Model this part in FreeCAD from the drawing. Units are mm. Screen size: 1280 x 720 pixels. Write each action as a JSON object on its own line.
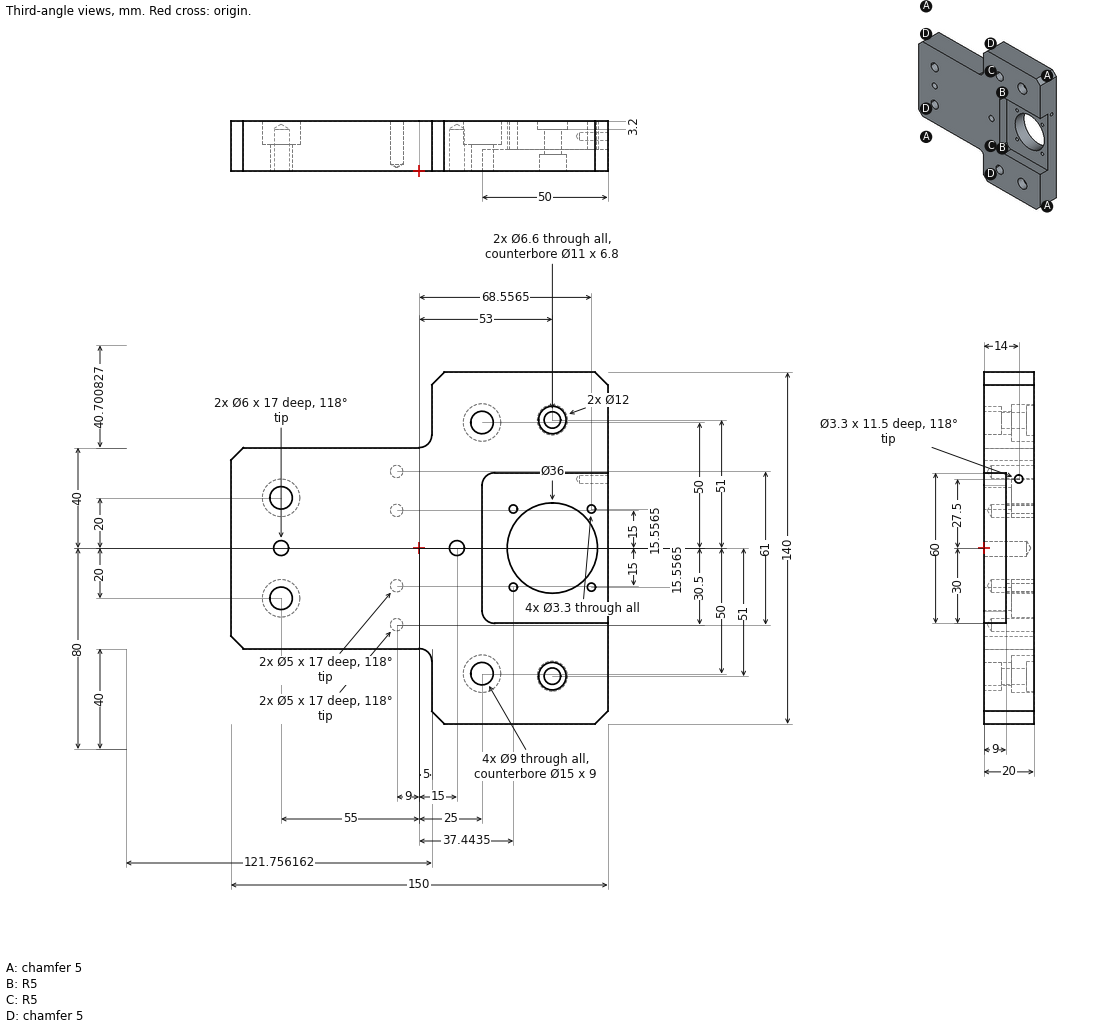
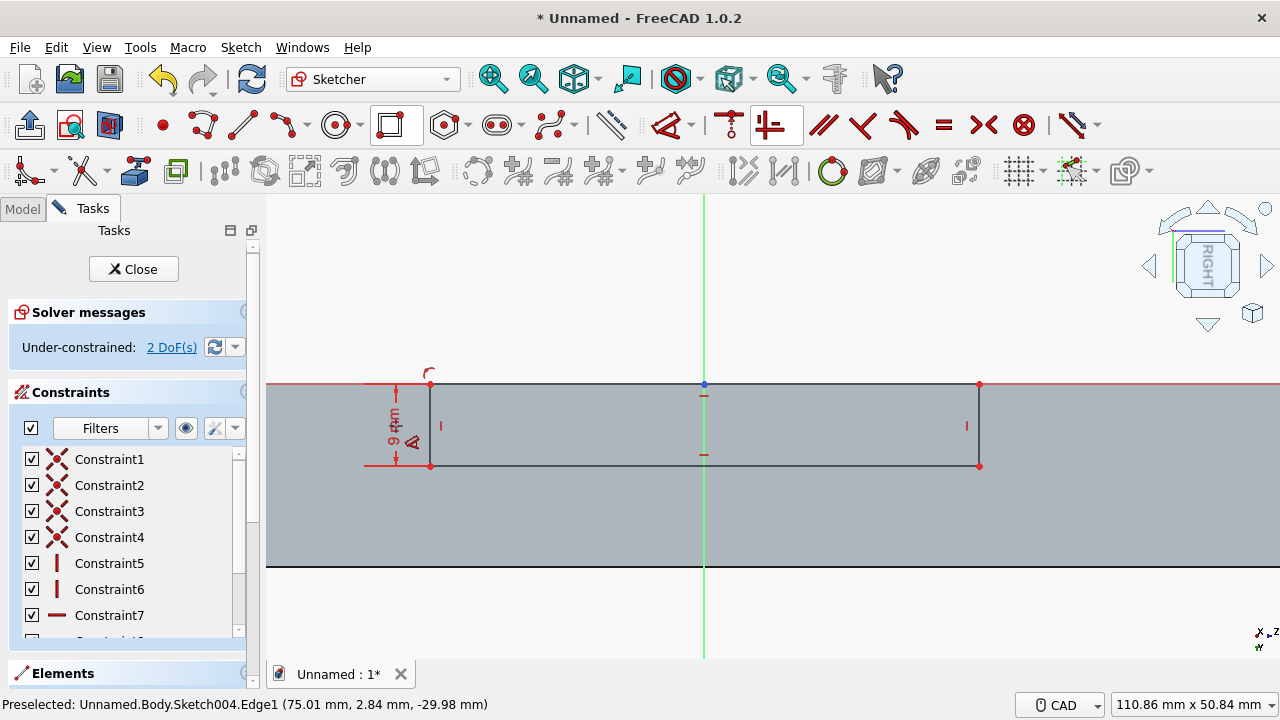
{"action": "left_click", "coordinate": [595, 466]}
{"action": "left_click", "coordinate": [578, 500]}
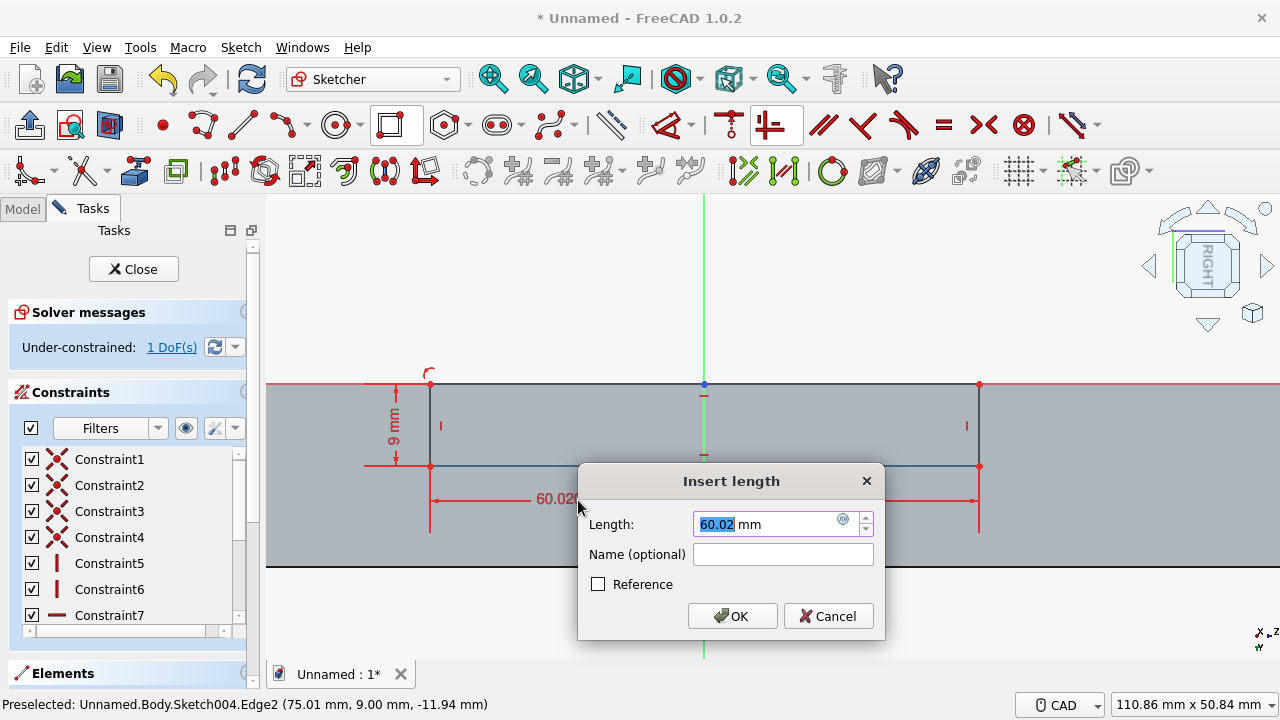
{"action": "type", "text": "60"}
{"action": "key", "text": "Return"}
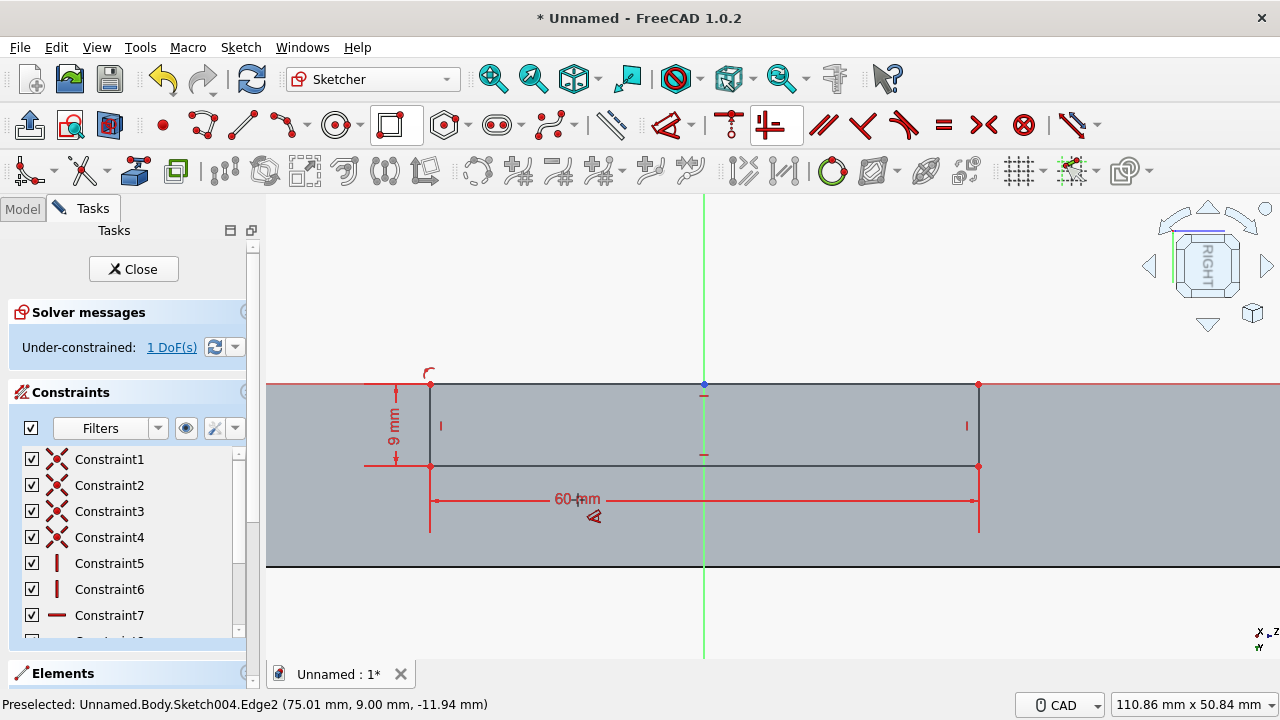
{"action": "left_click", "coordinate": [430, 384]}
{"action": "left_click", "coordinate": [567, 350]}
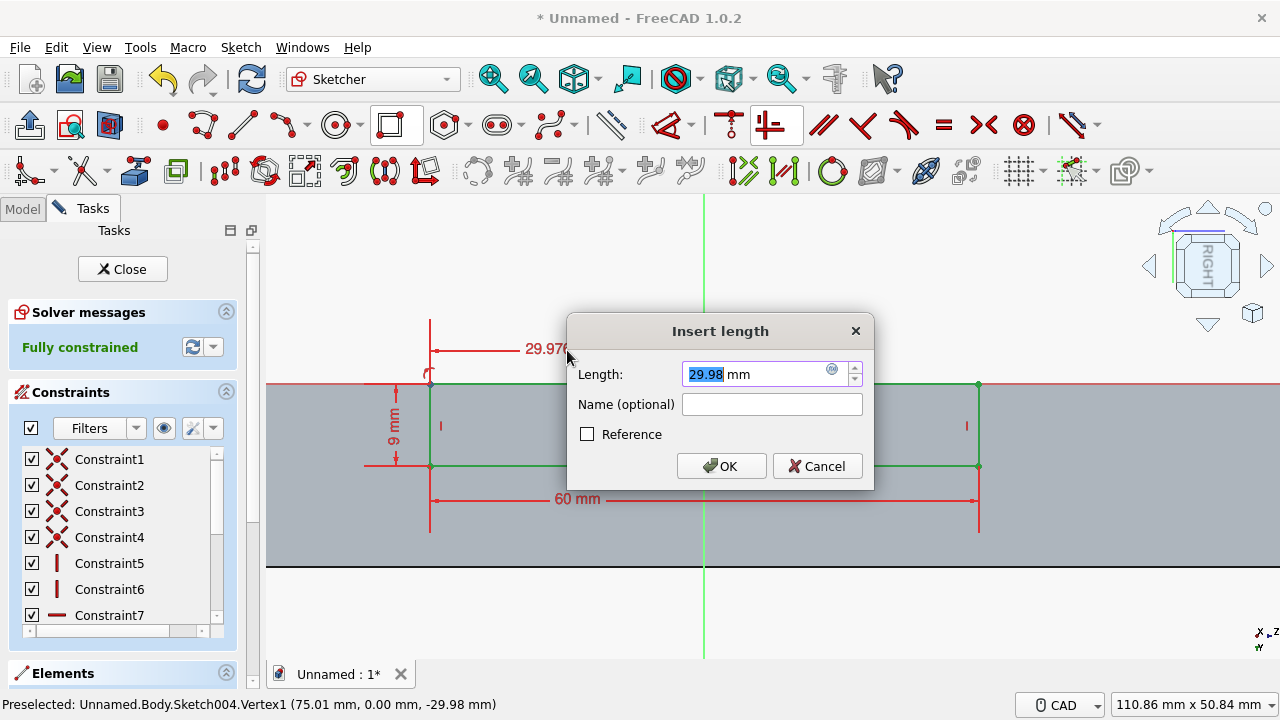
{"action": "type", "text": "30"}
{"action": "key", "text": "Return"}
{"action": "key", "text": "Escape"}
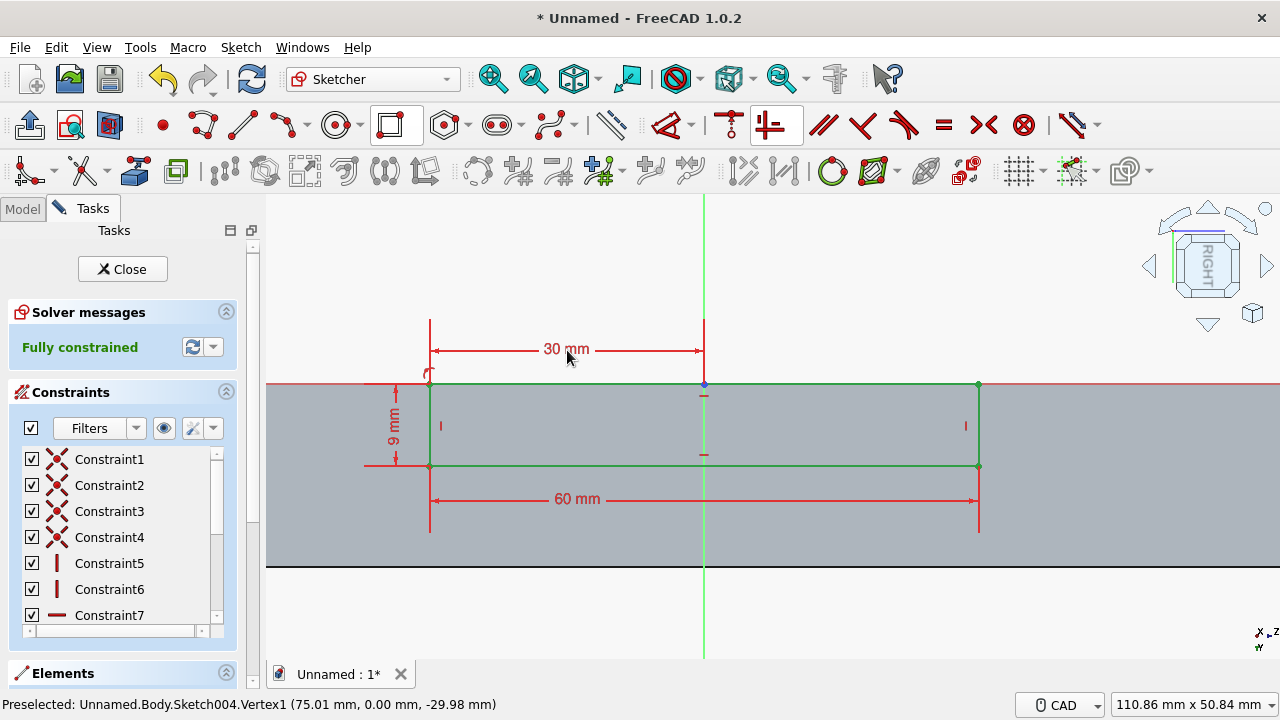
{"action": "left_click", "coordinate": [123, 269]}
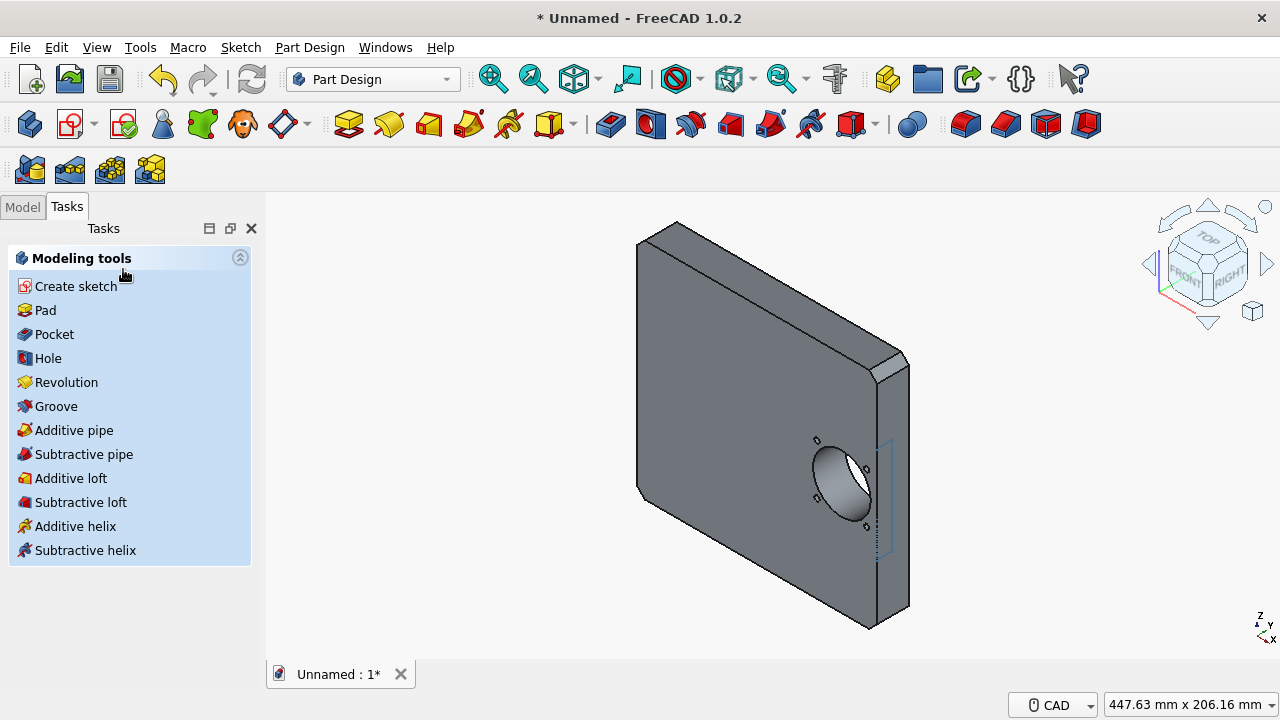
{"action": "left_click", "coordinate": [612, 124]}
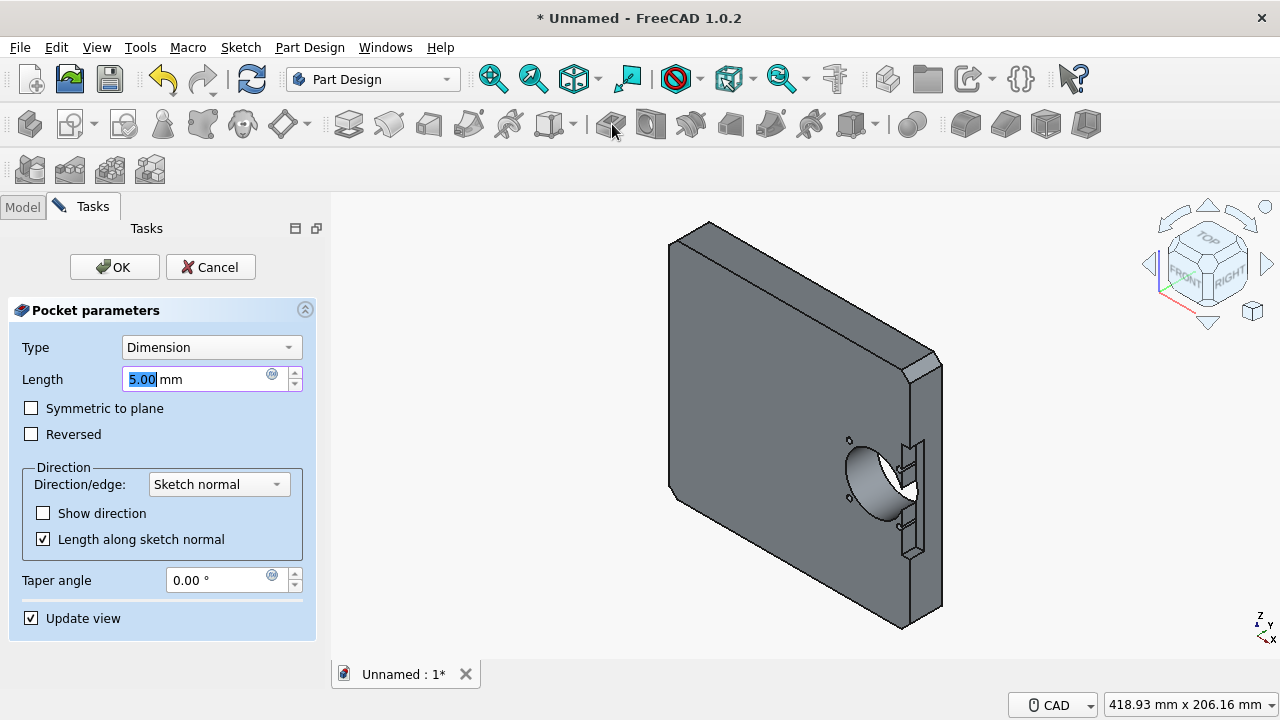
{"action": "type", "text": "50"}
{"action": "key", "text": "Tab"}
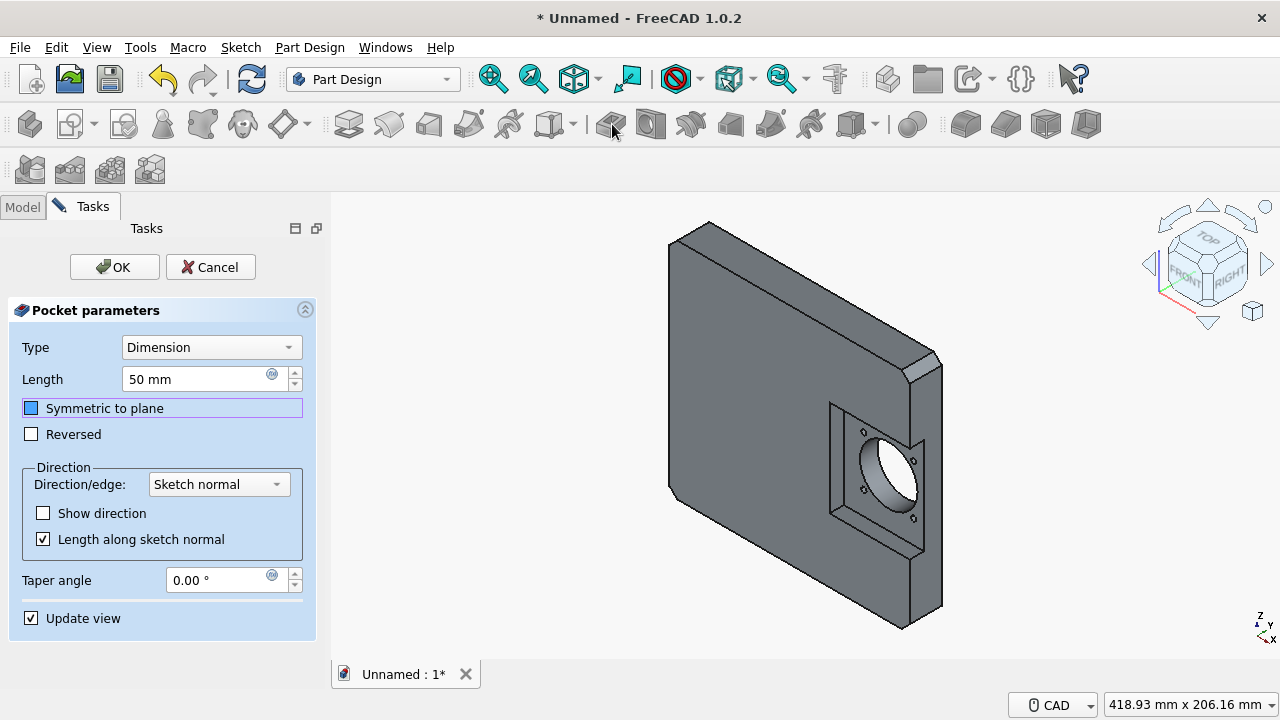
{"action": "left_click", "coordinate": [115, 267]}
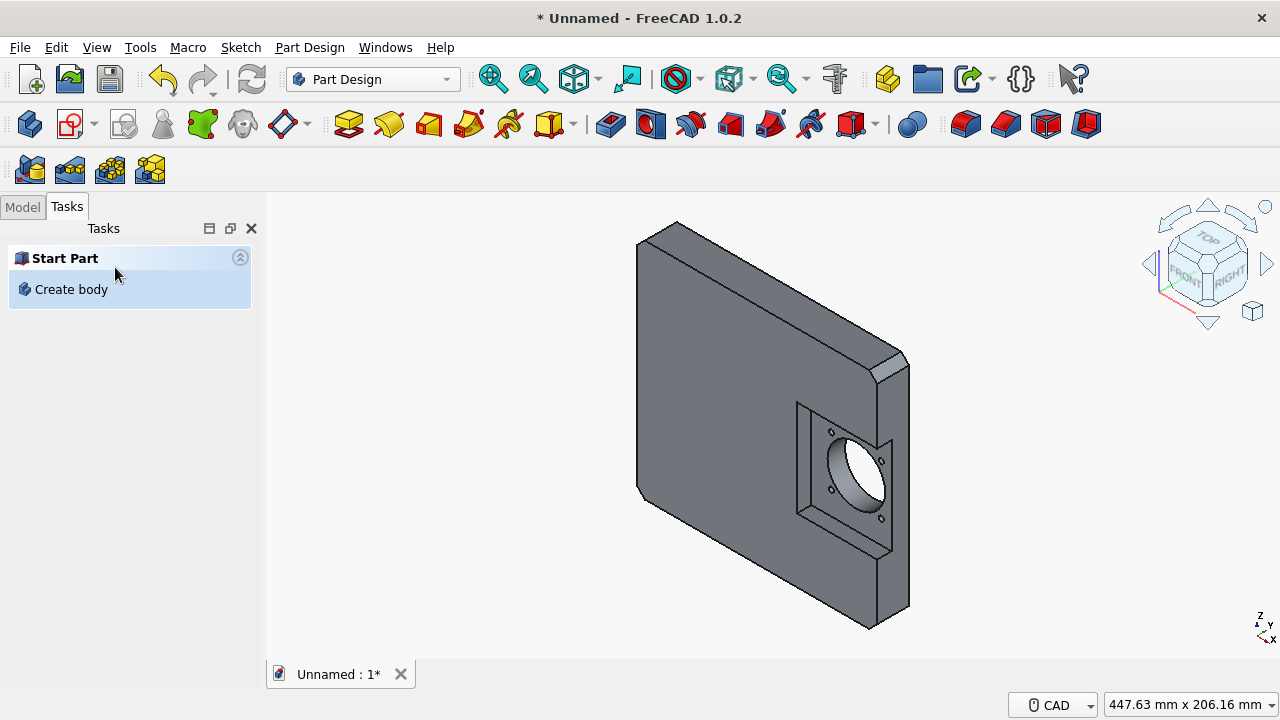
{"action": "left_click", "coordinate": [893, 597]}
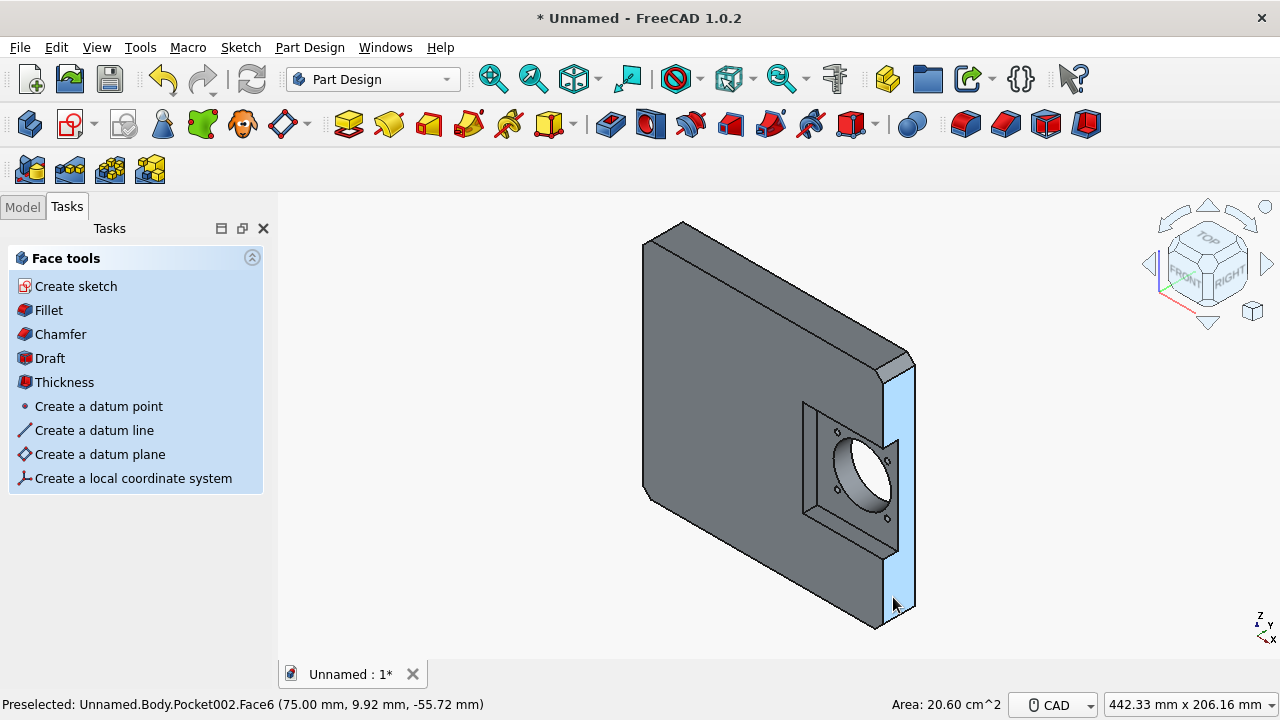
{"action": "left_click", "coordinate": [70, 124]}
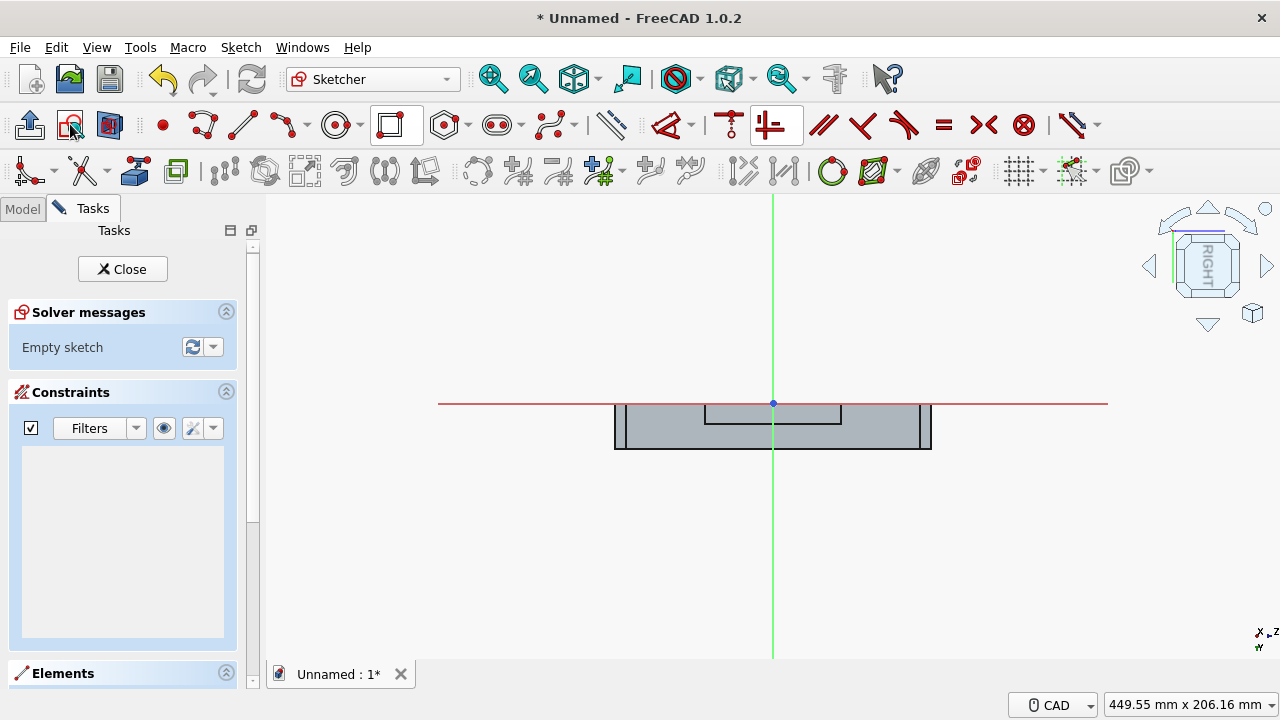
{"action": "scroll", "coordinate": [842, 436], "scroll_direction": "up", "scroll_amount": 15}